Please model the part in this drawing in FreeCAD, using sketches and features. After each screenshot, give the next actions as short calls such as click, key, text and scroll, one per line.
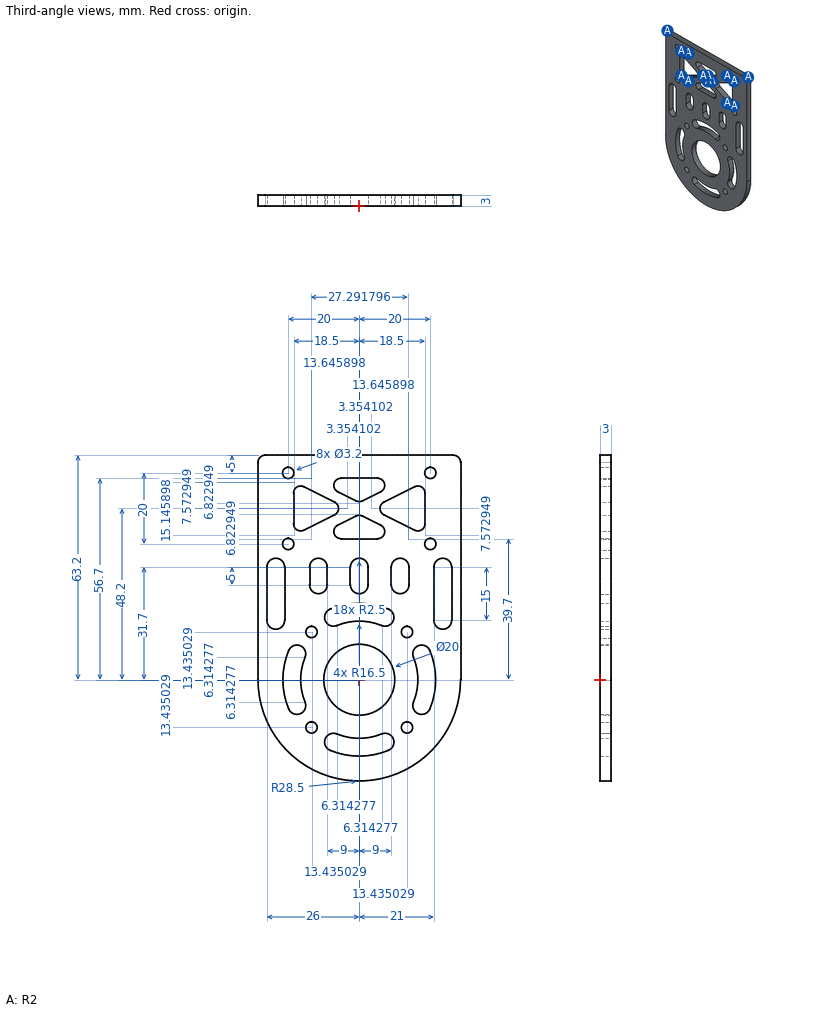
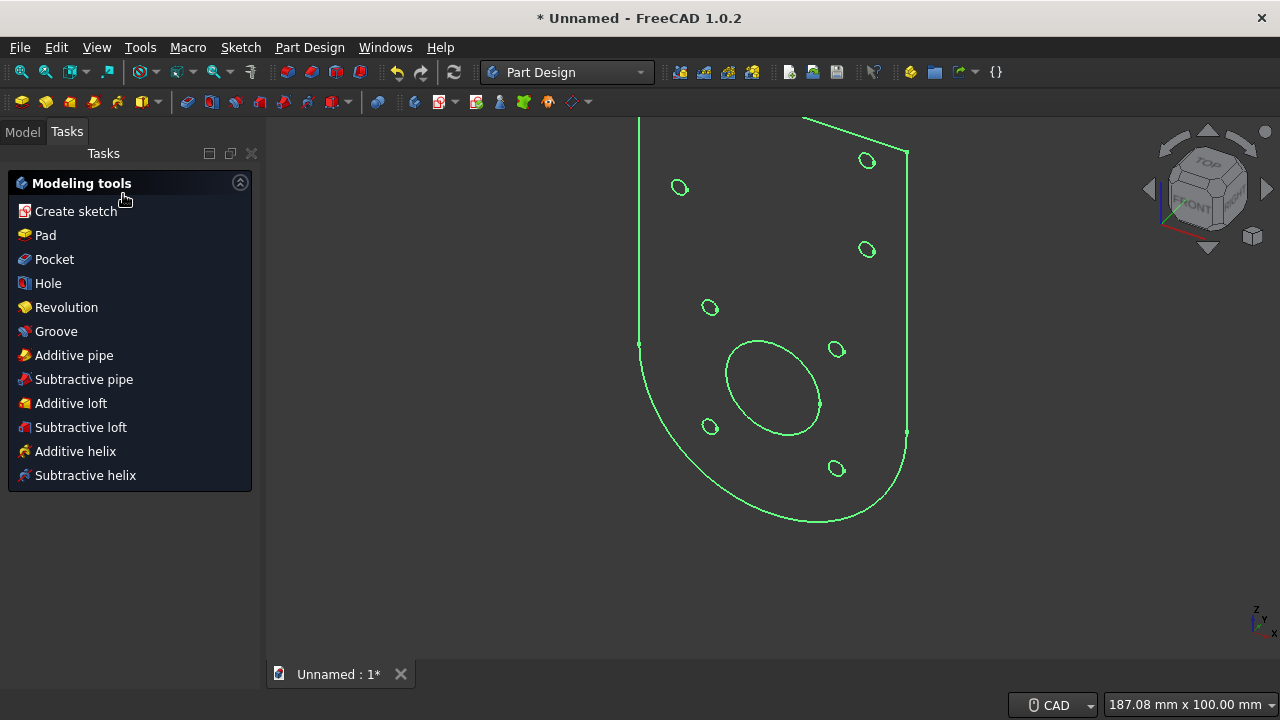
click(22, 102)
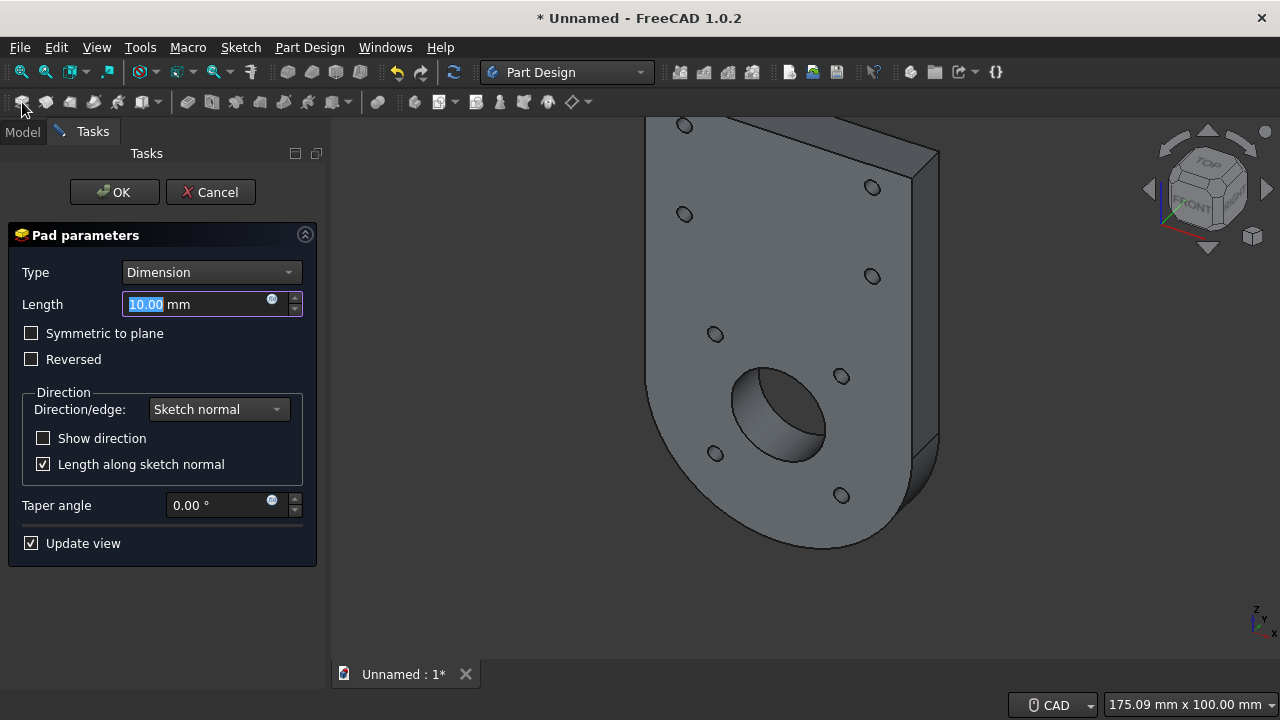
text(3)
key(Tab)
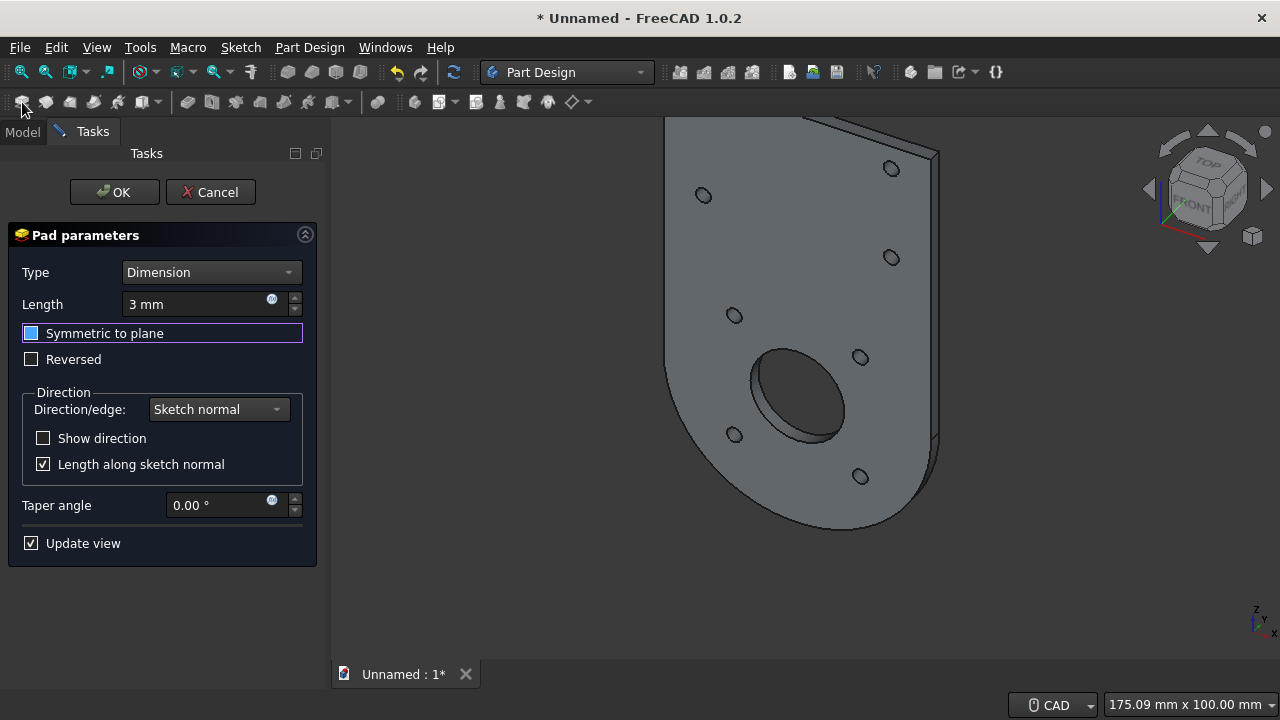
click(30, 359)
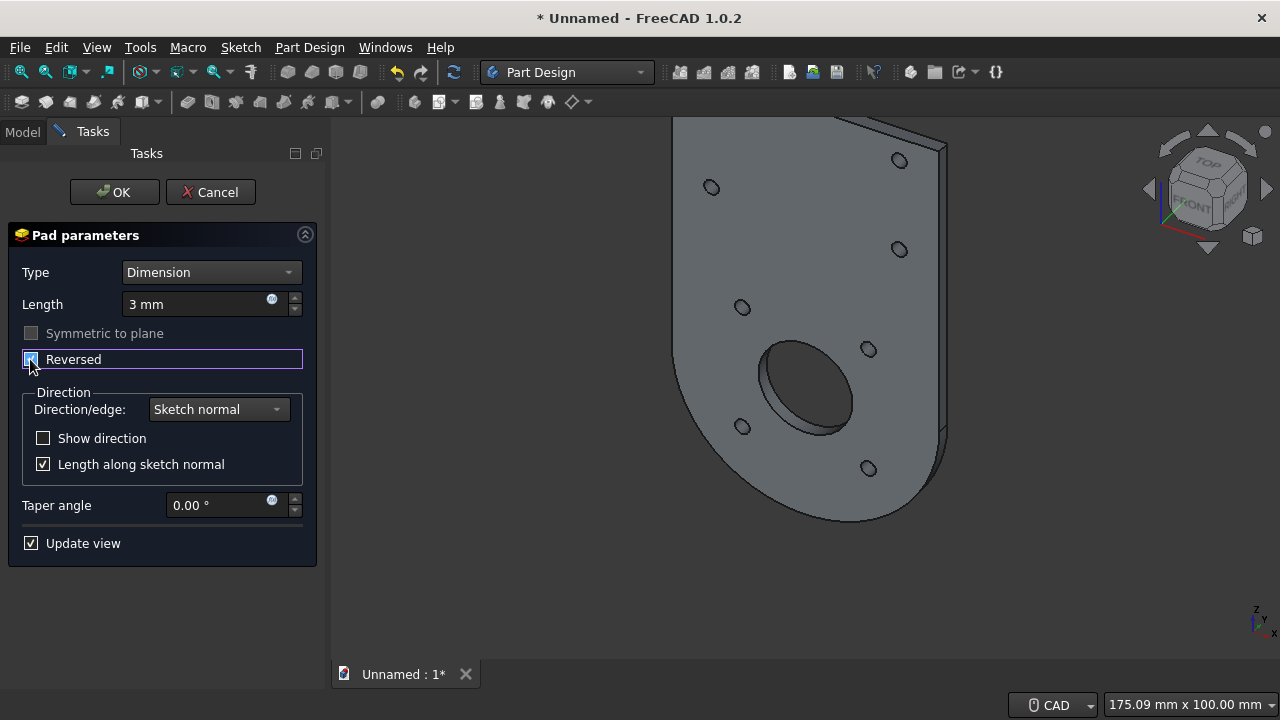
click(115, 192)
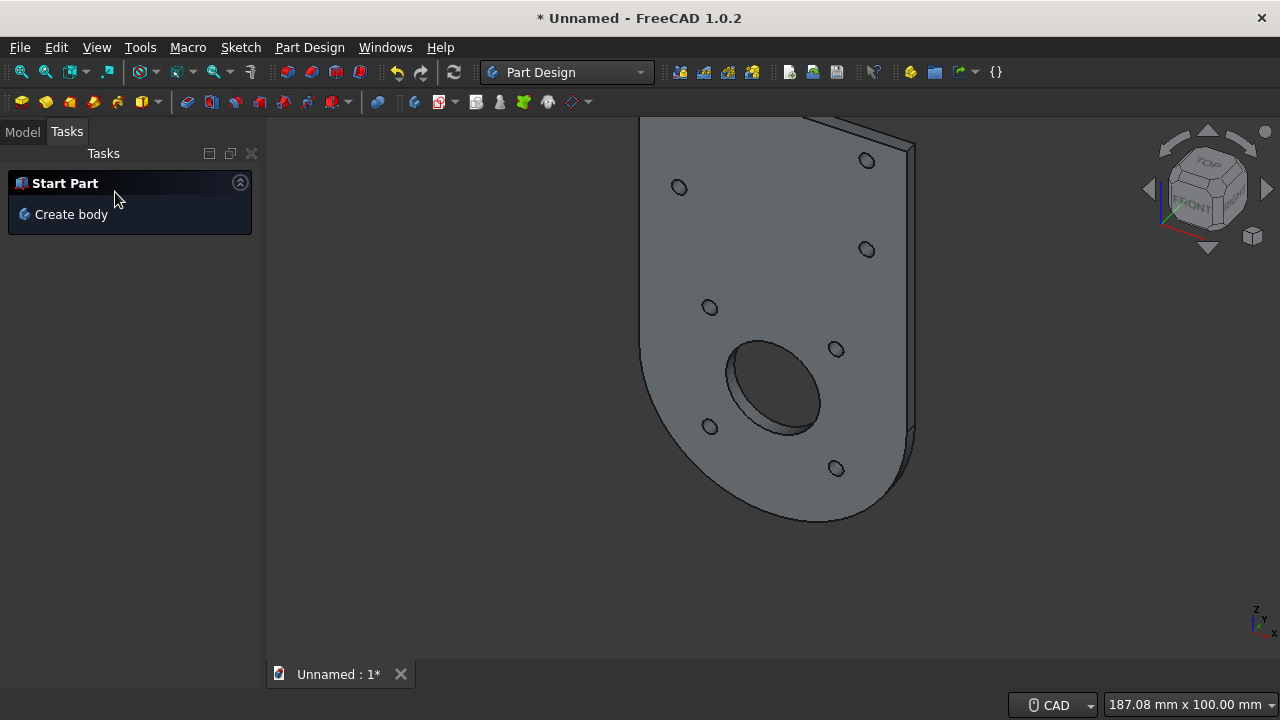
key(v)
key(f)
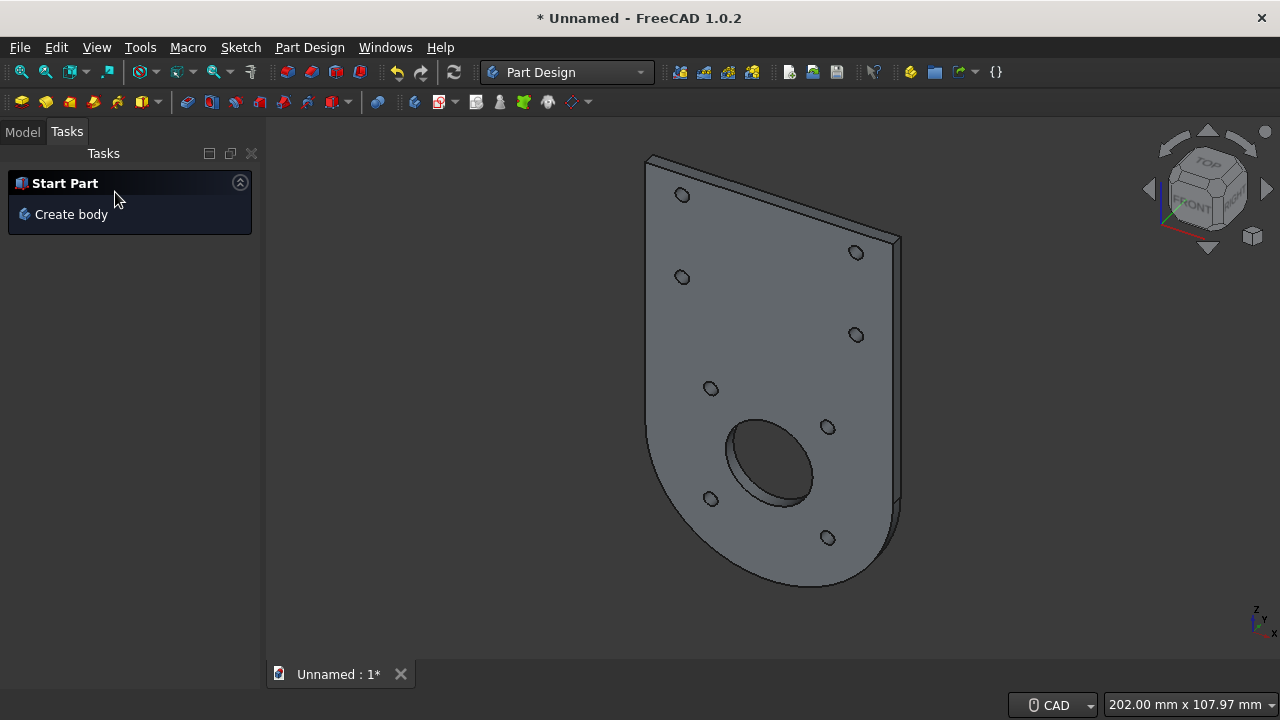
key(4)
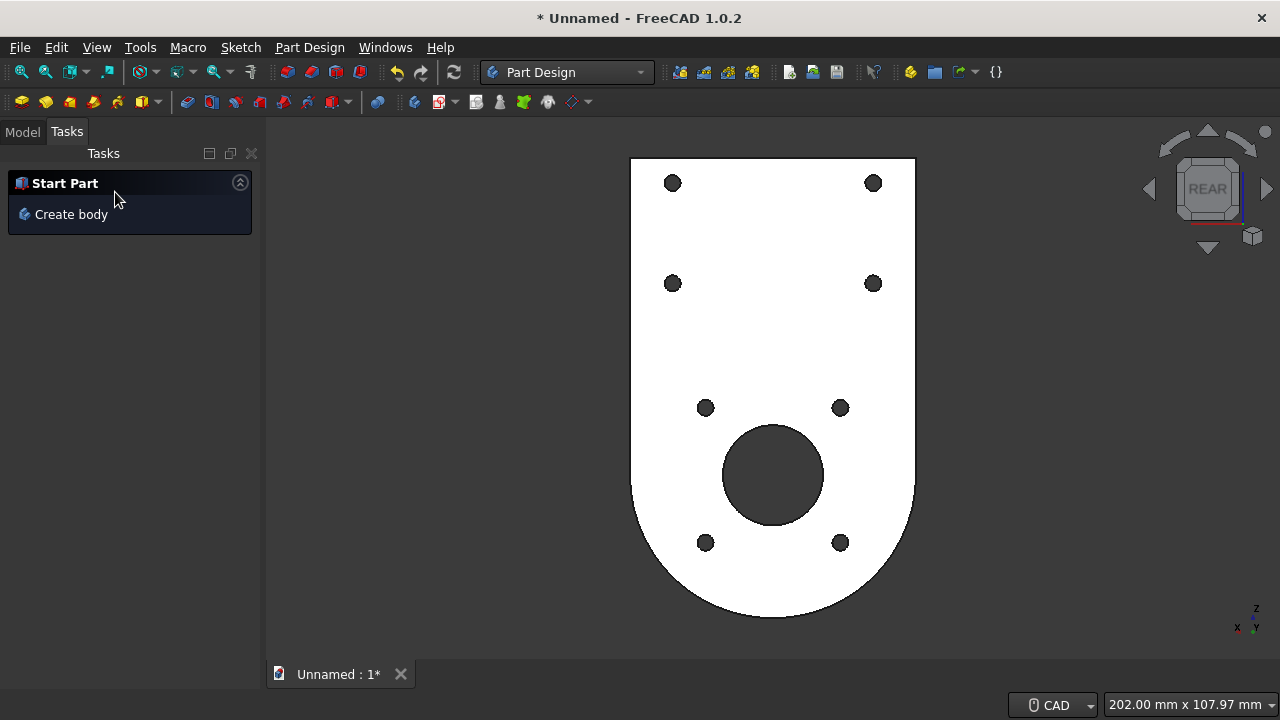
click(773, 321)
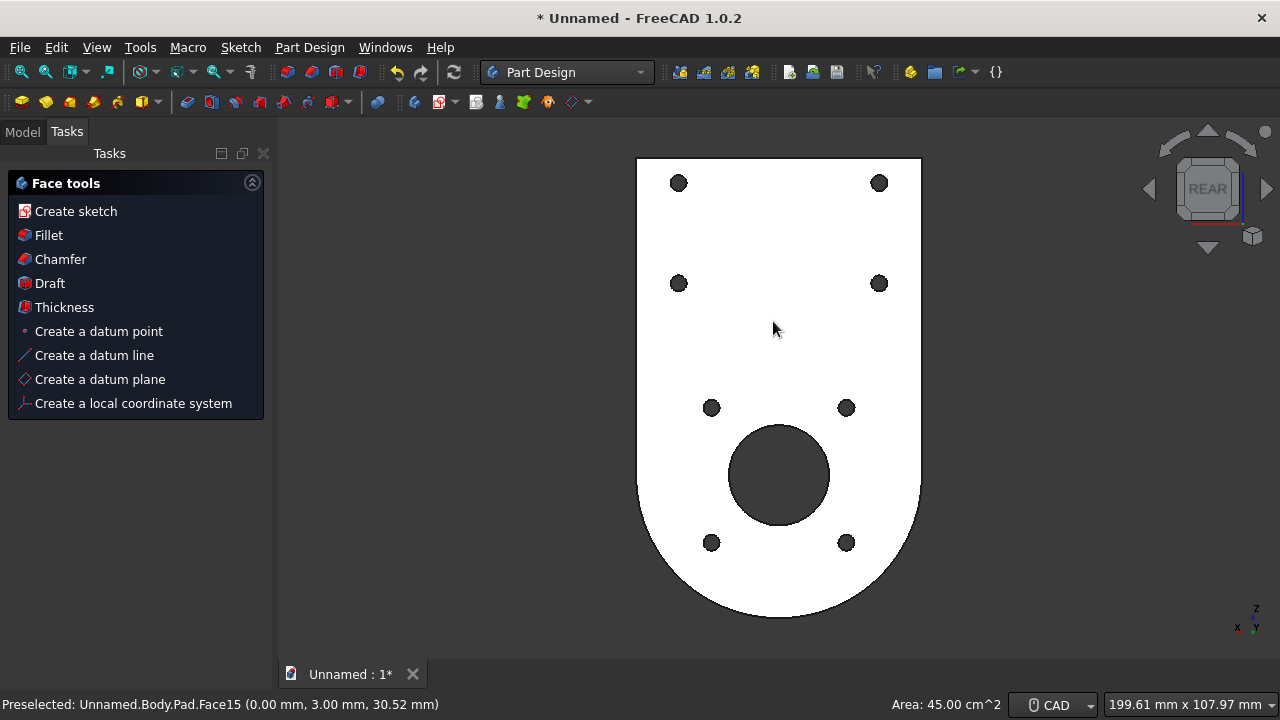
click(440, 102)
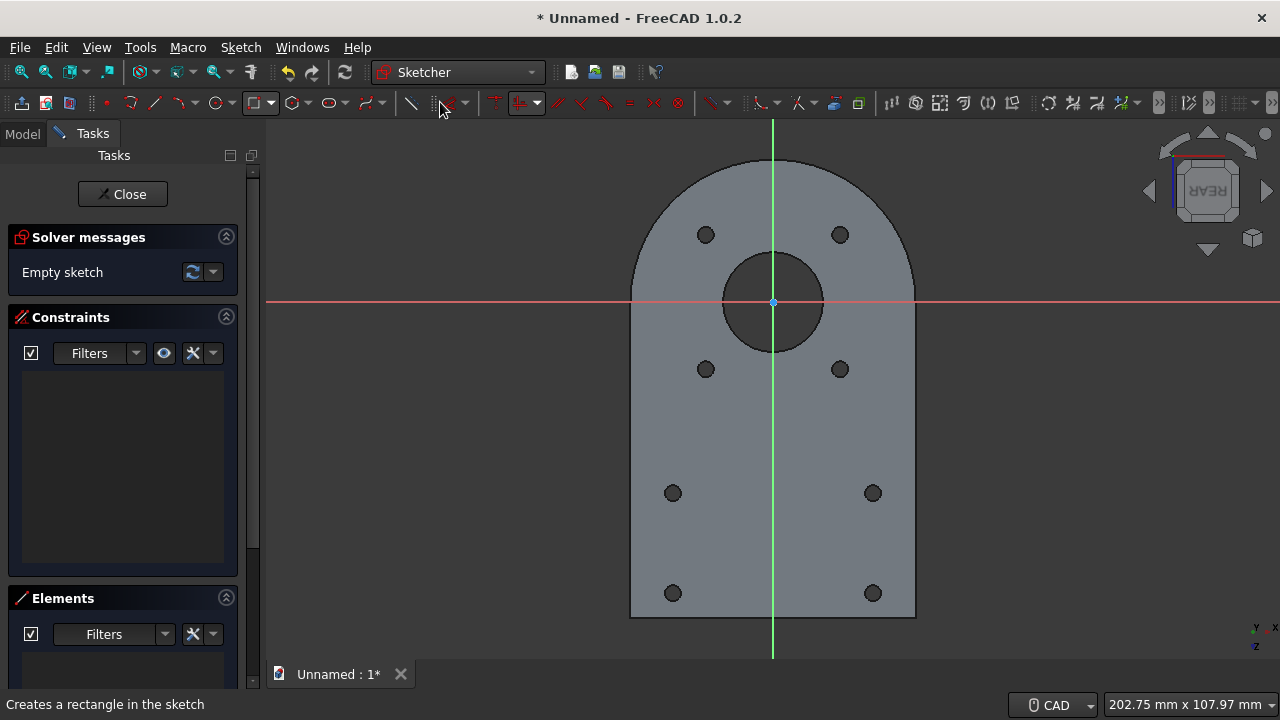
key(g)
key(m)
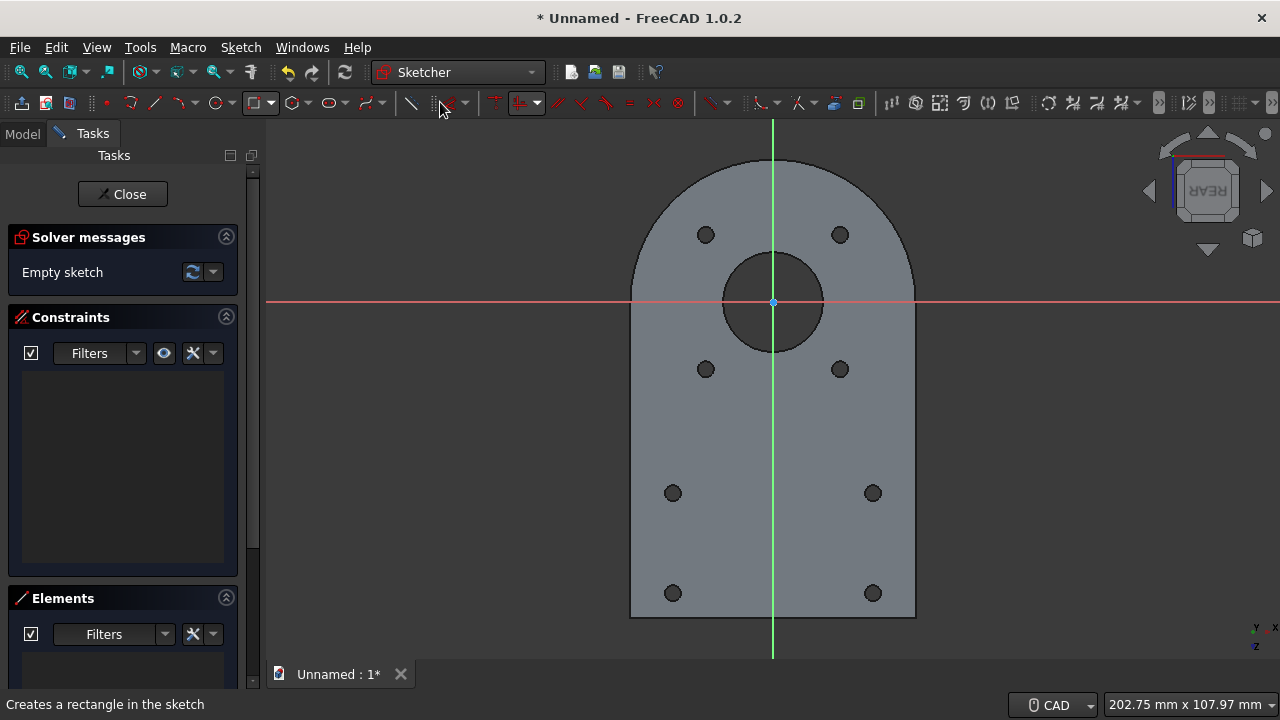
click(680, 505)
click(680, 581)
click(756, 543)
click(680, 506)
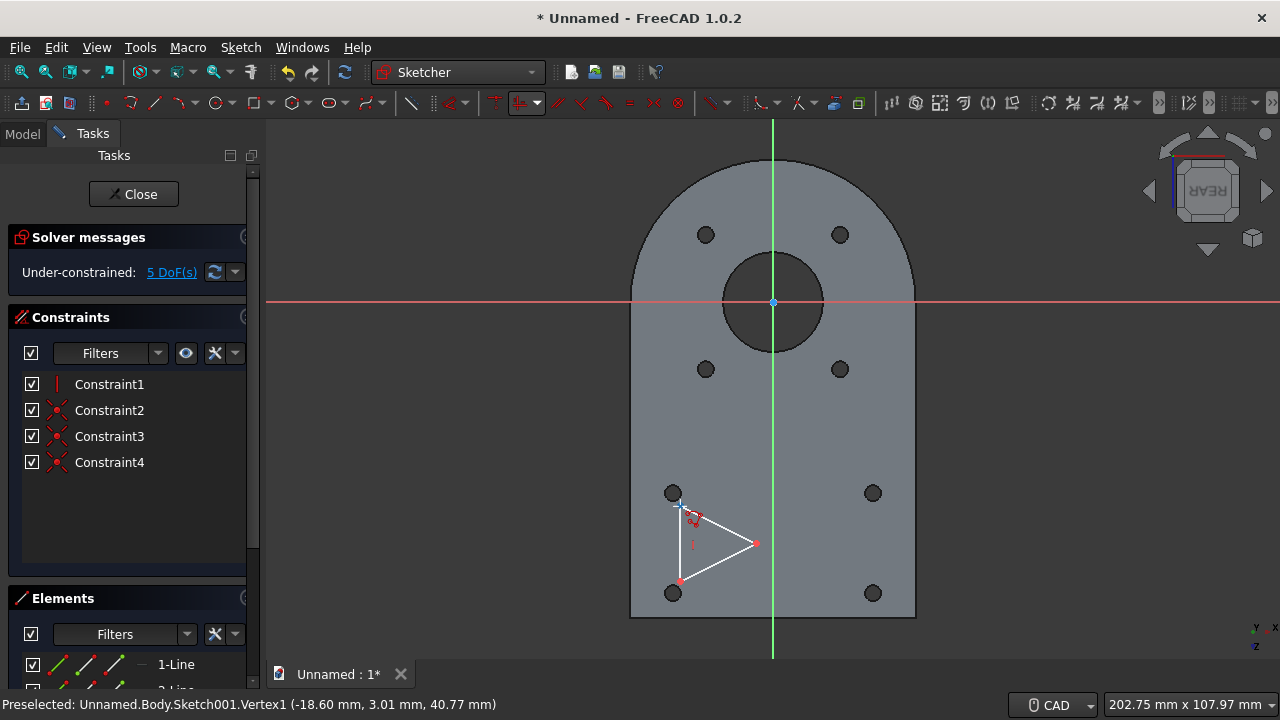
click(841, 501)
click(705, 501)
click(773, 535)
click(841, 502)